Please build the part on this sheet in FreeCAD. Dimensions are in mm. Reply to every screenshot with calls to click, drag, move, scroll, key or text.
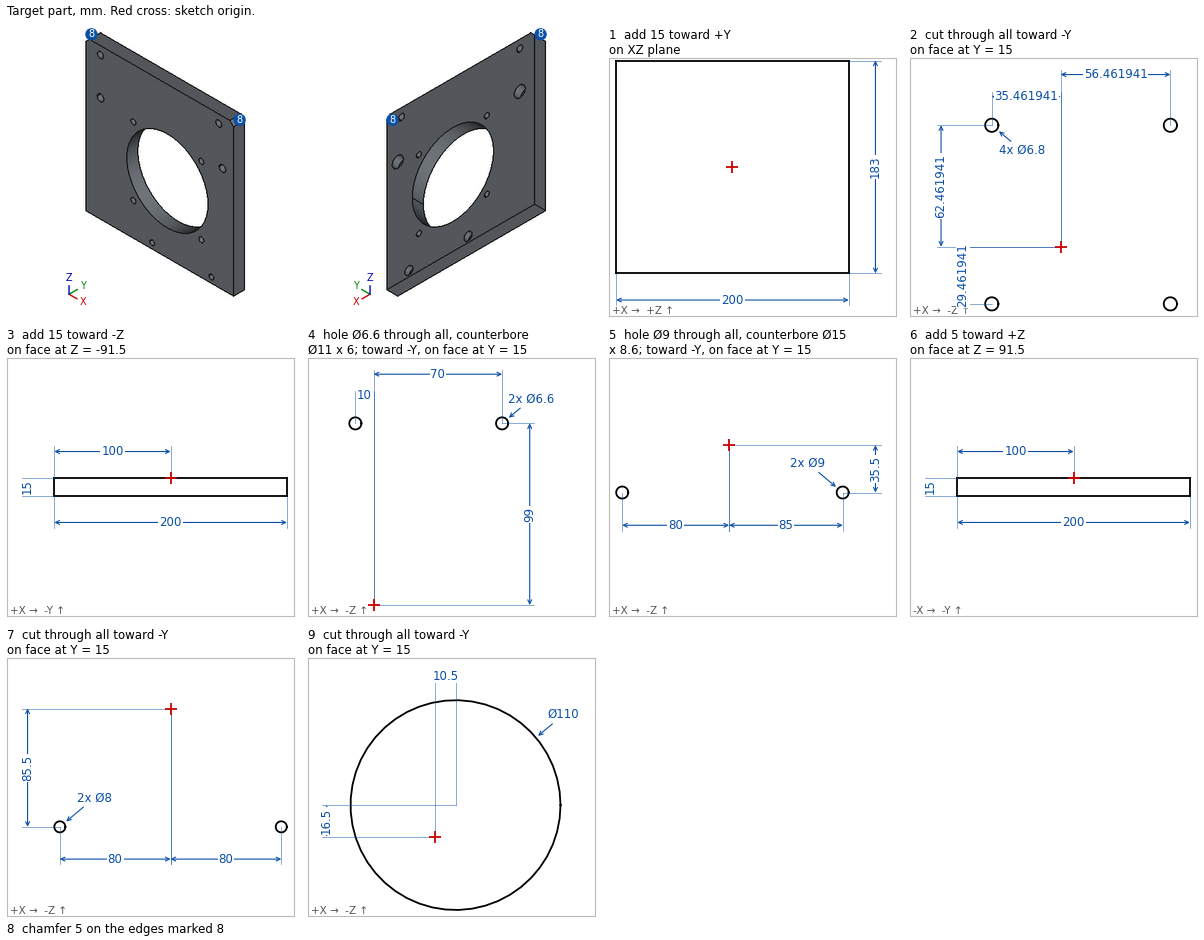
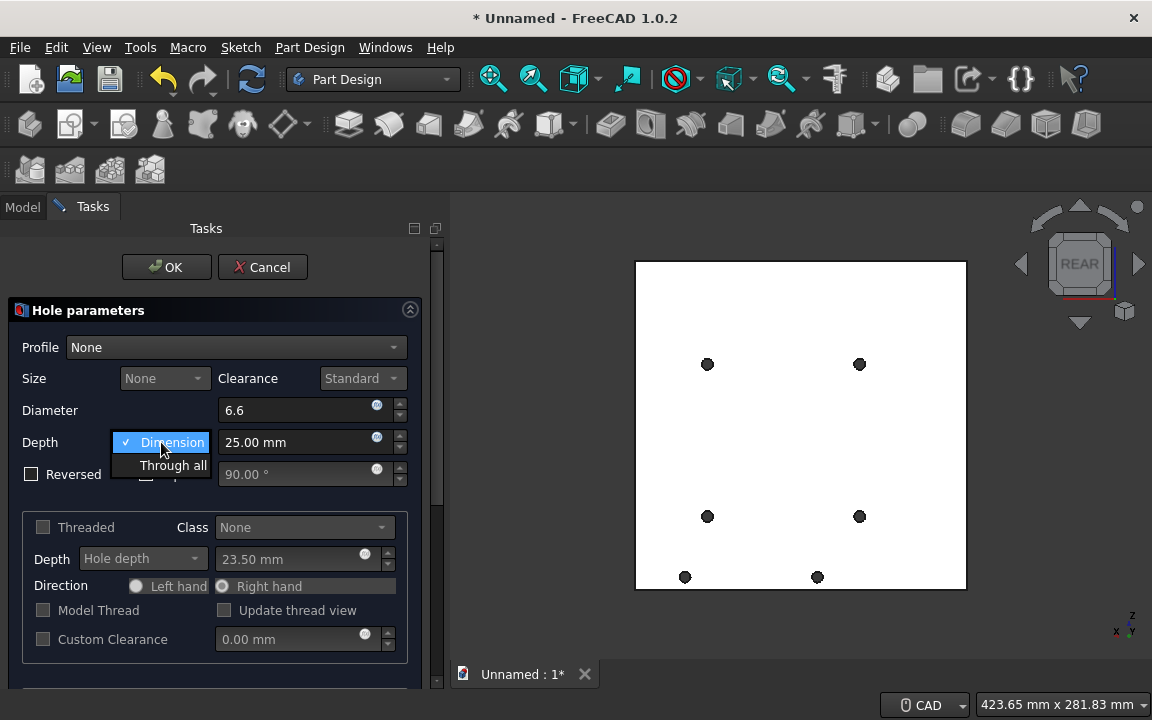
click(160, 466)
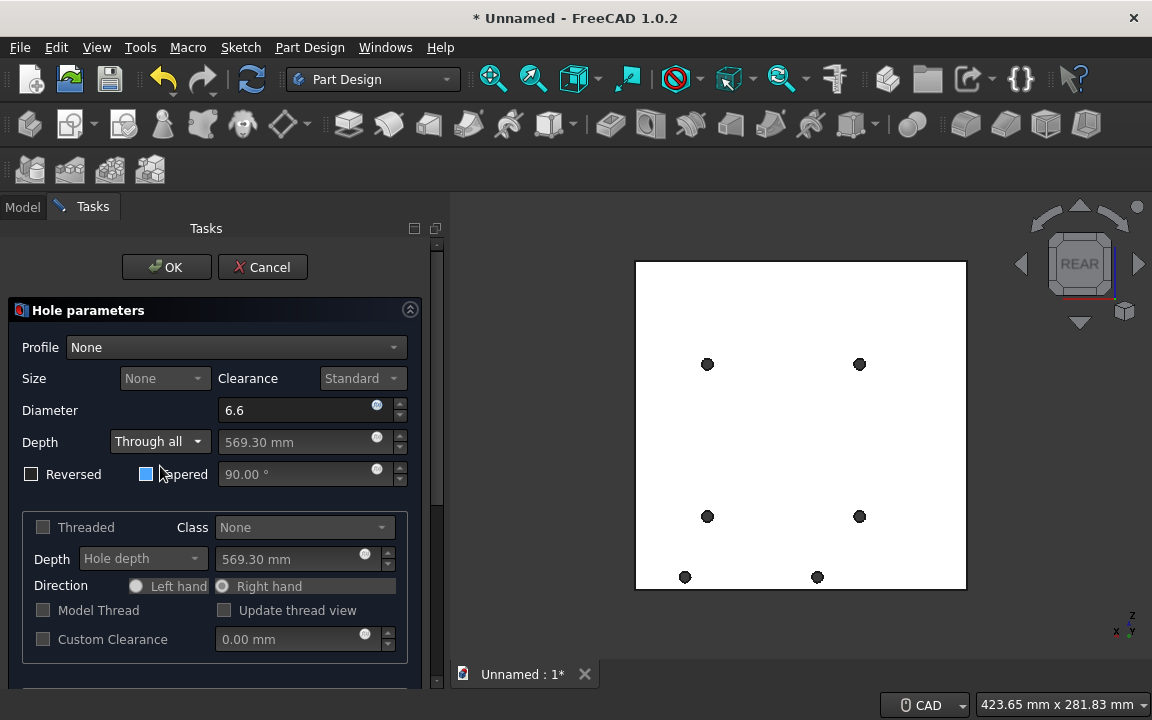
scroll(437, 463, down, 2)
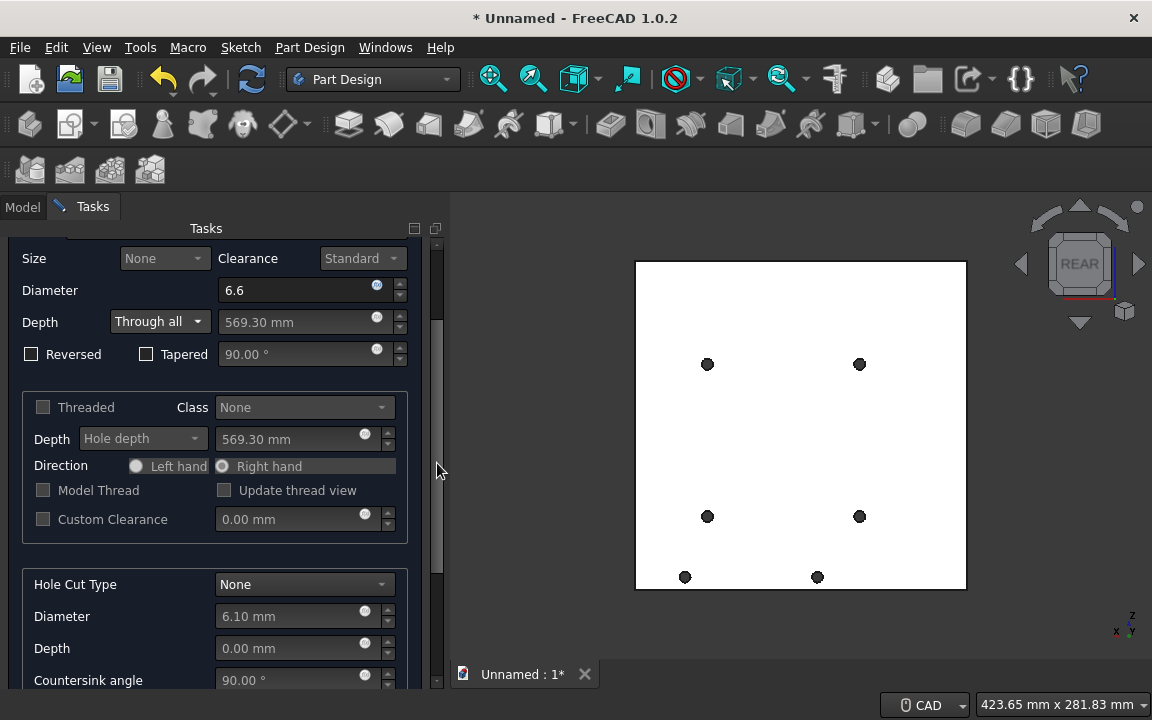
click(306, 584)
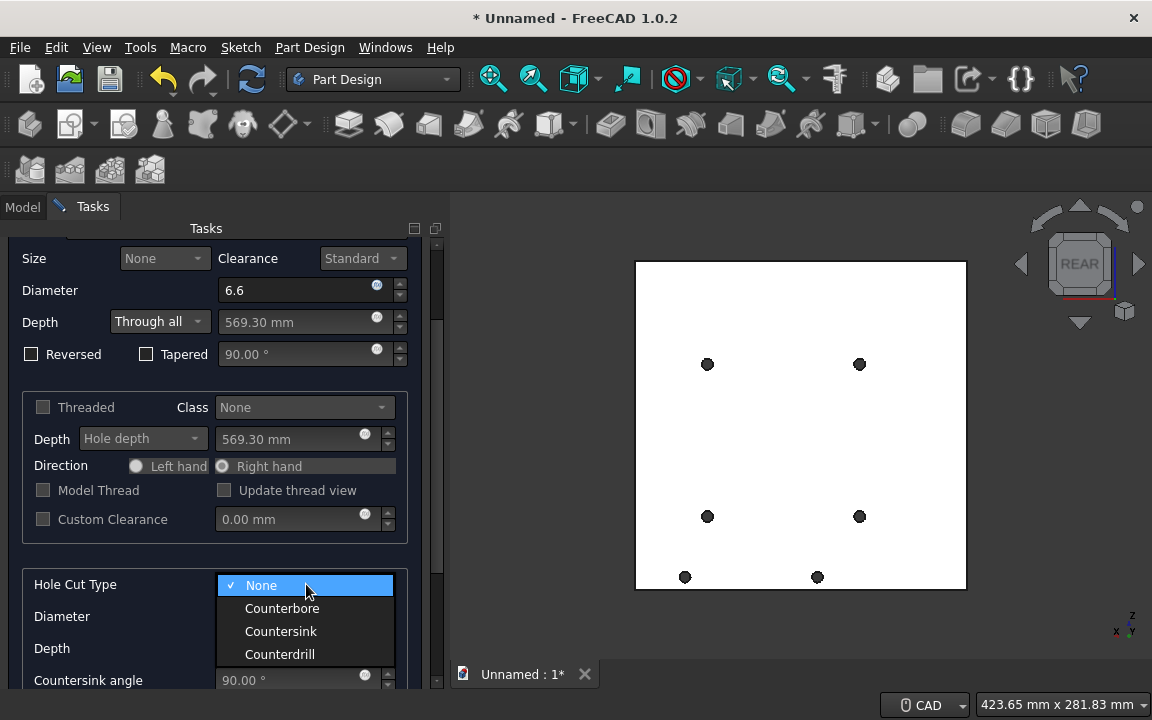
click(304, 608)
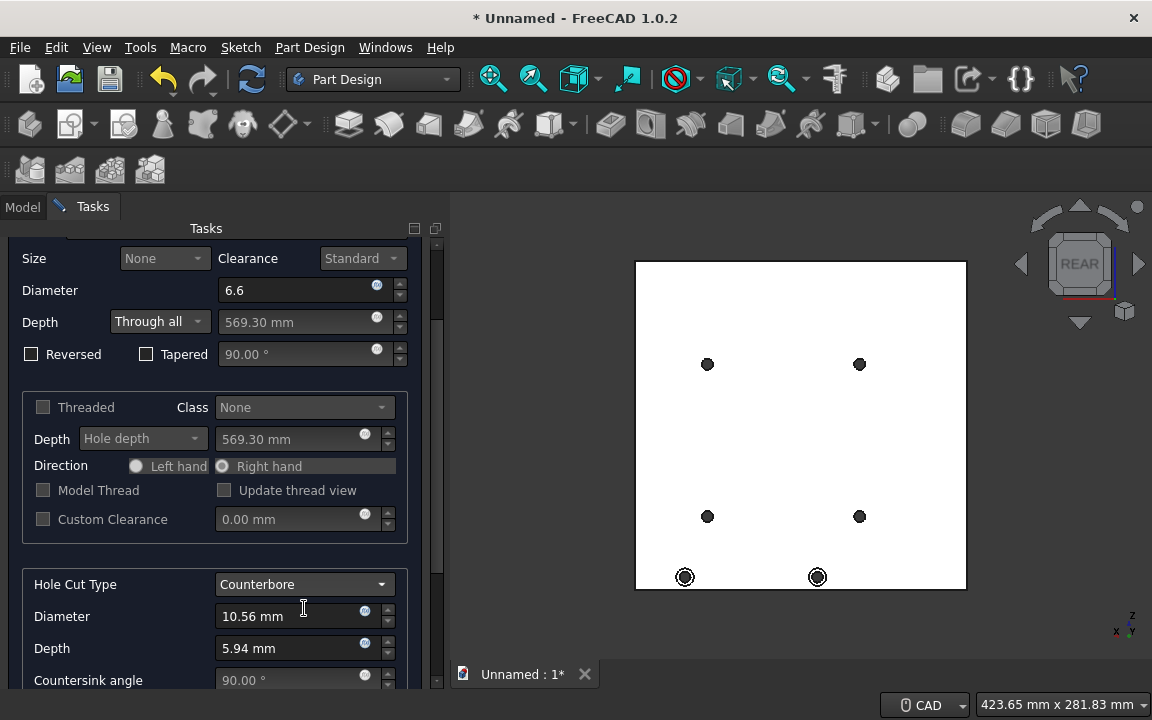
triple_click(298, 616)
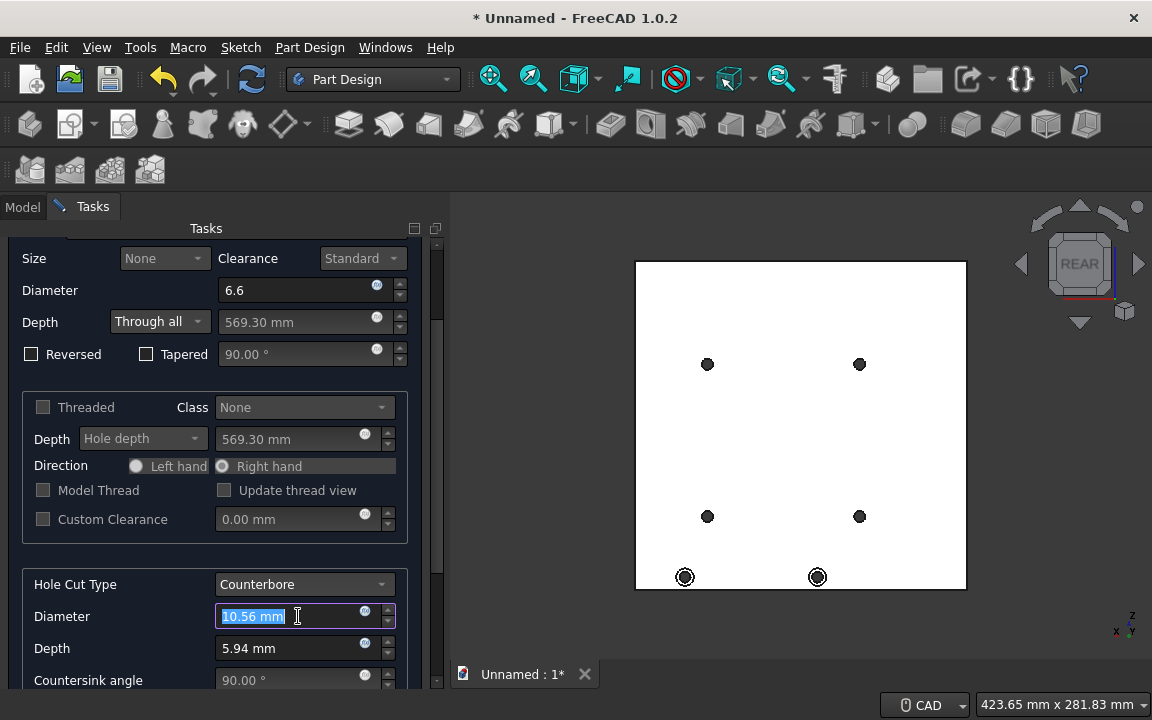
text(11)
key(Tab)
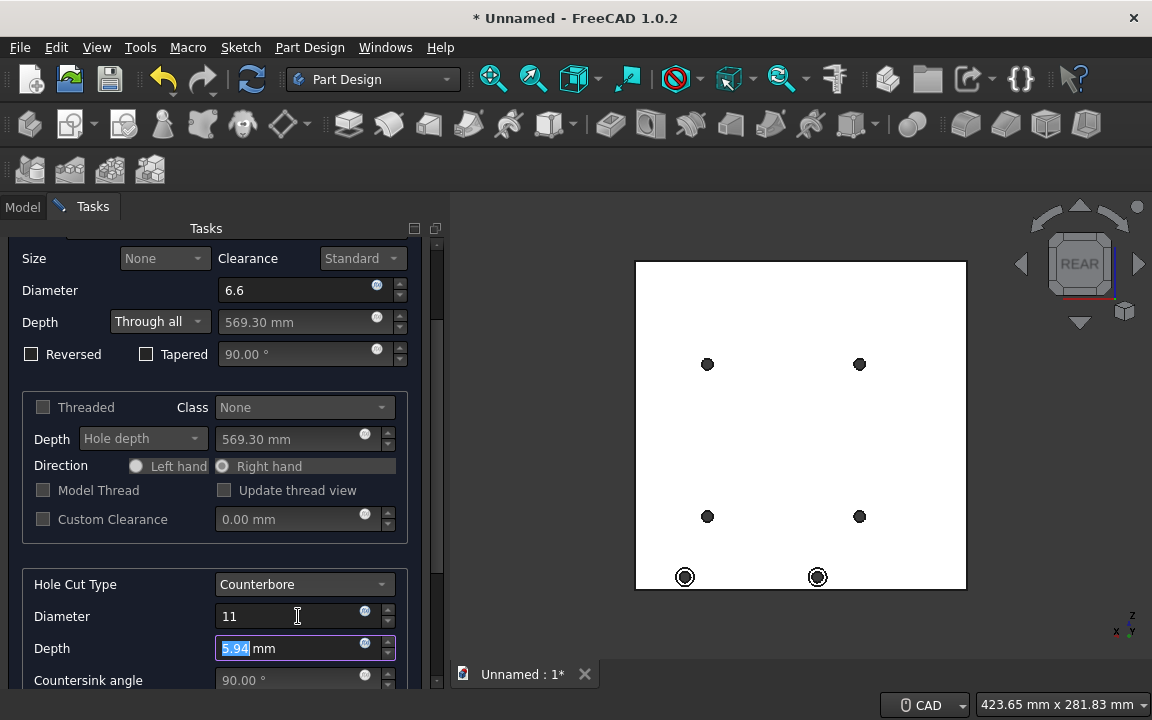
text(6)
key(Tab)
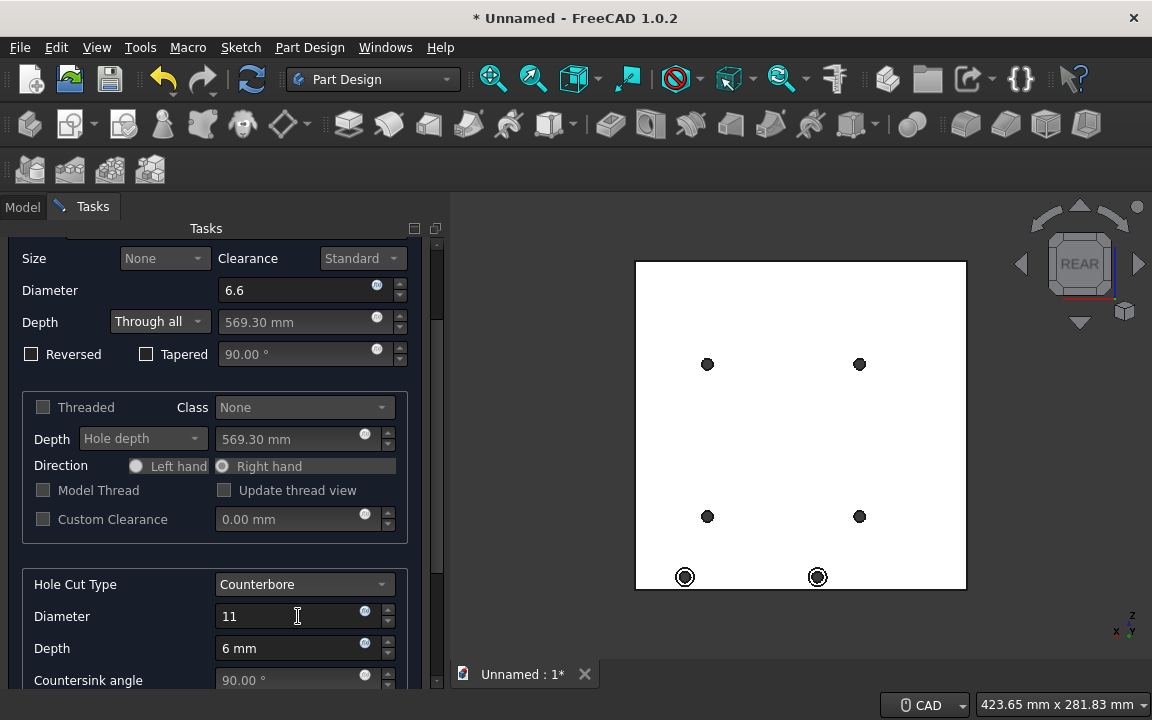
scroll(437, 463, up, 3)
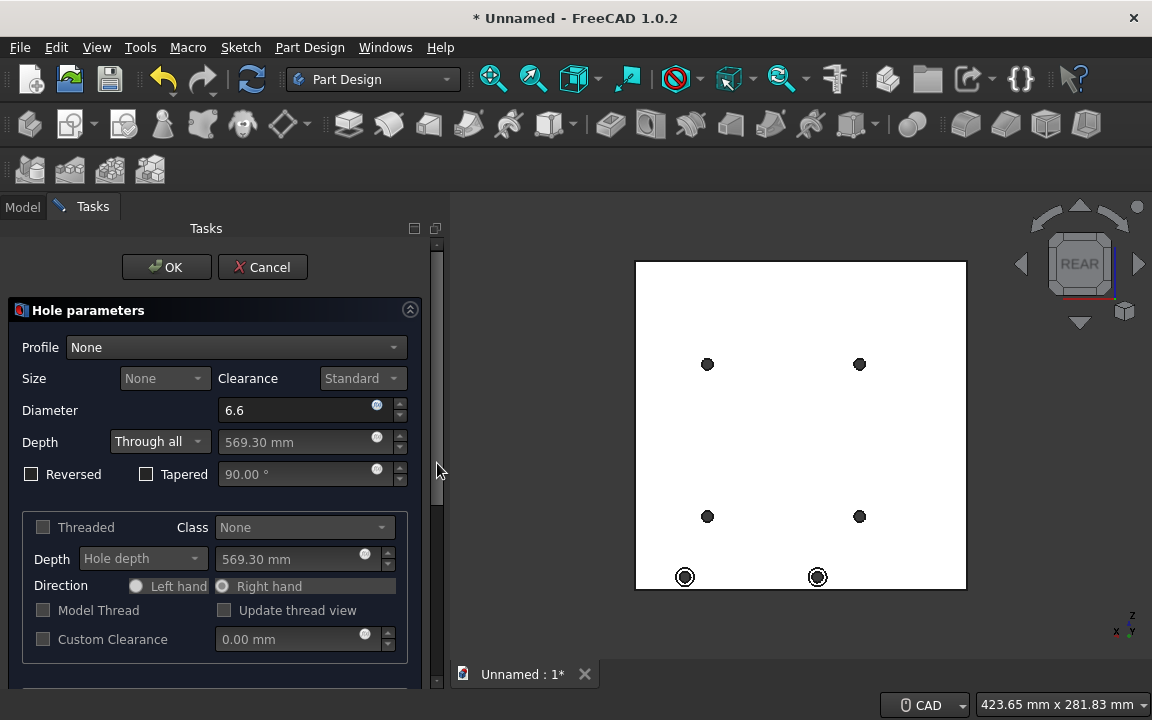
click(167, 267)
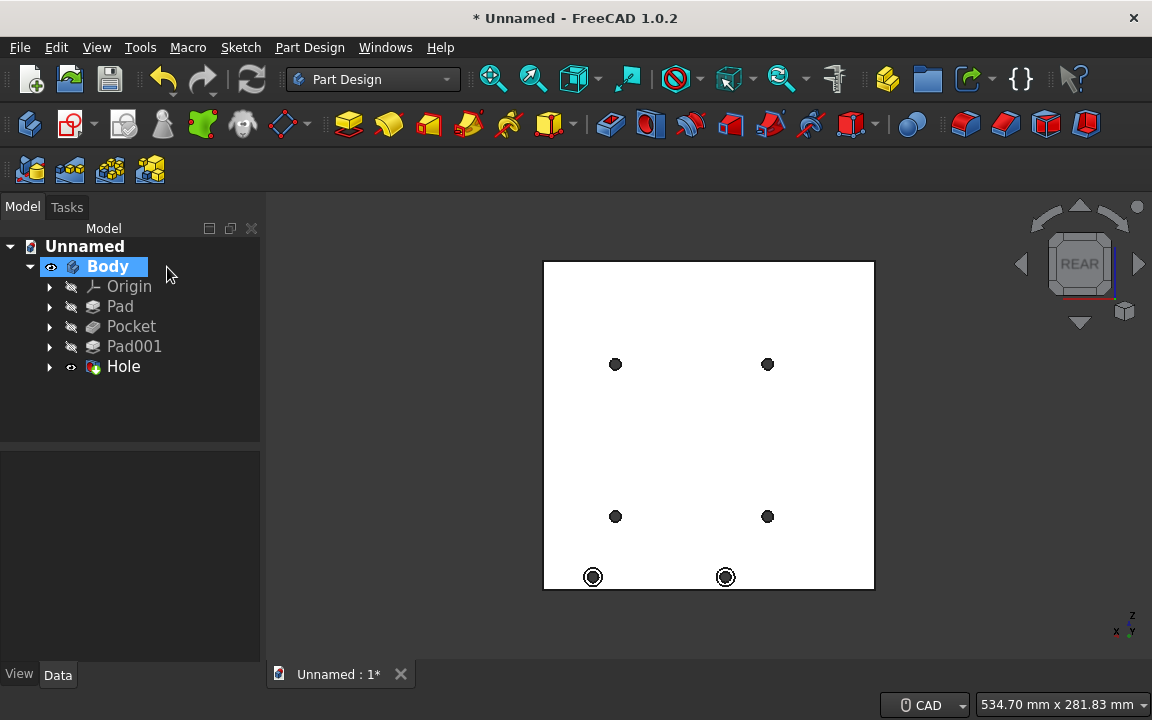
click(709, 424)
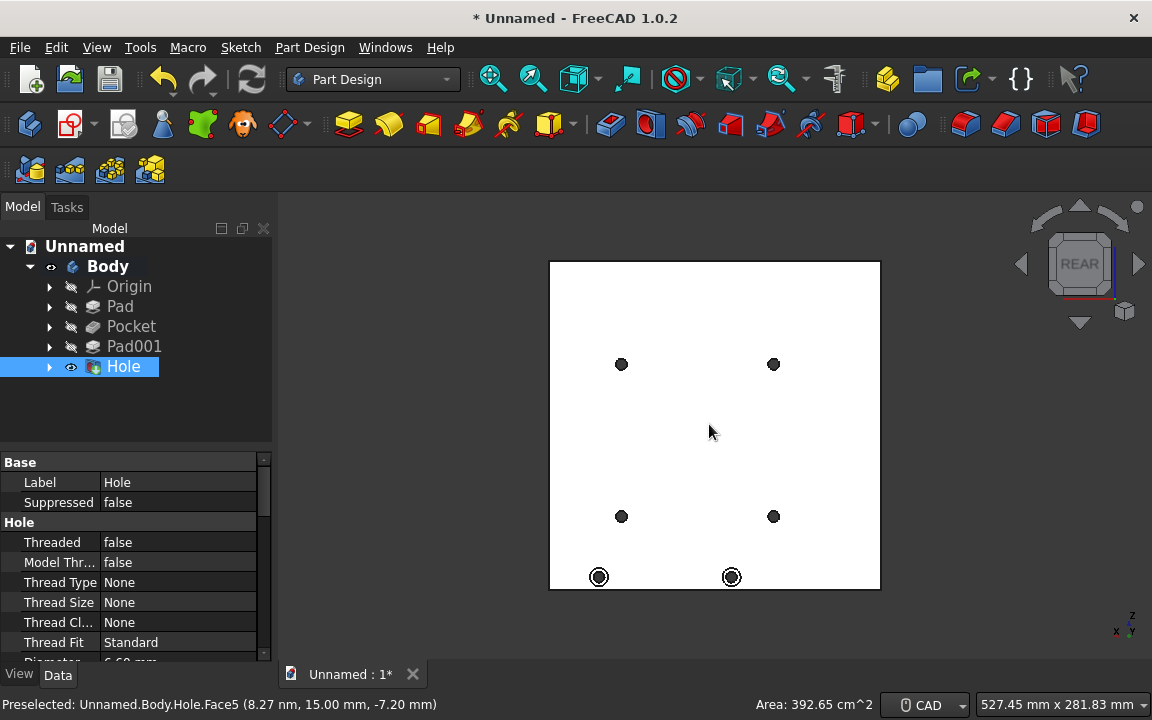
click(70, 124)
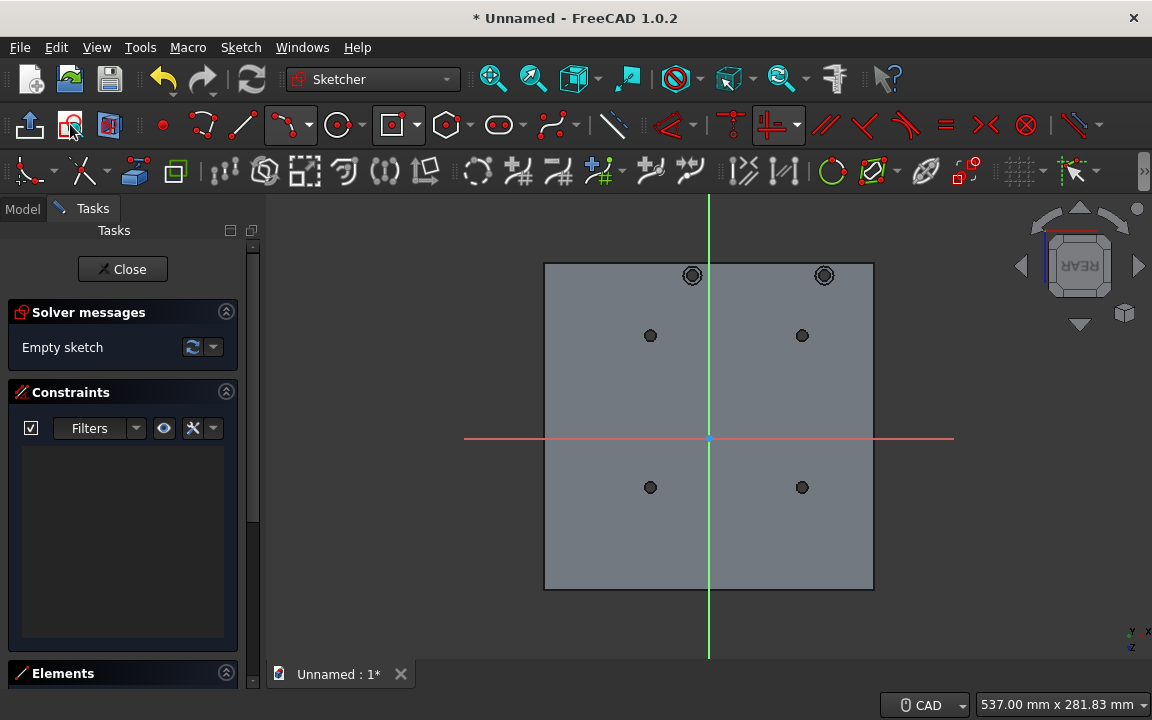
scroll(801, 527, up, 3)